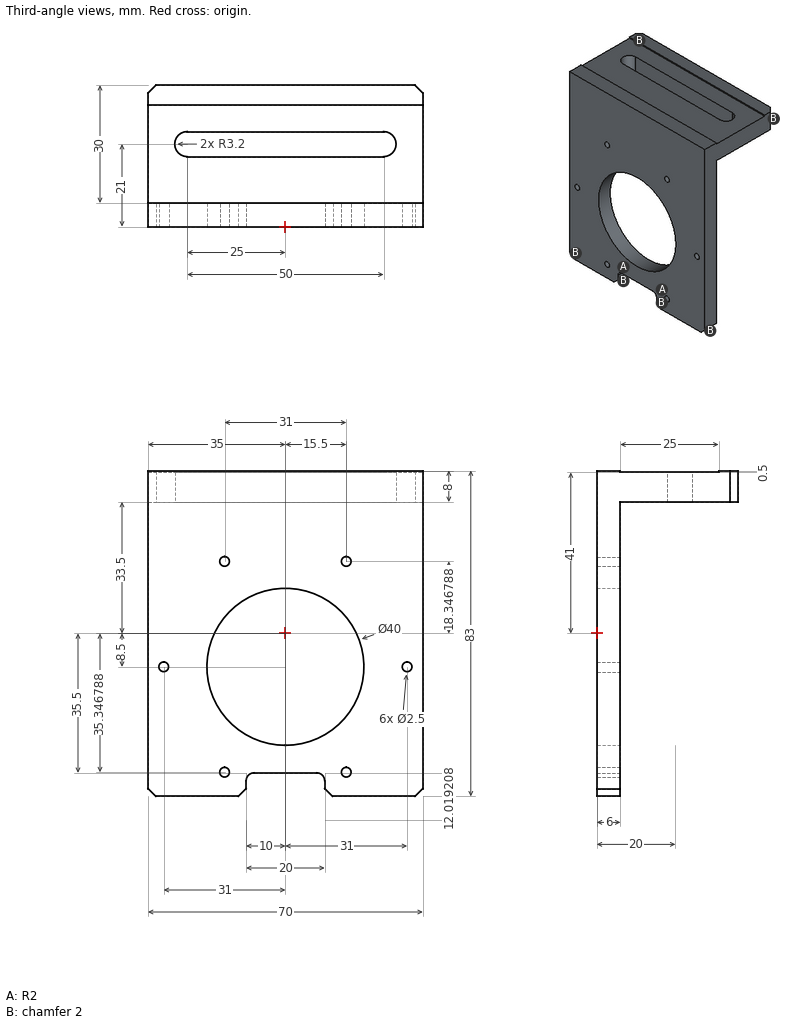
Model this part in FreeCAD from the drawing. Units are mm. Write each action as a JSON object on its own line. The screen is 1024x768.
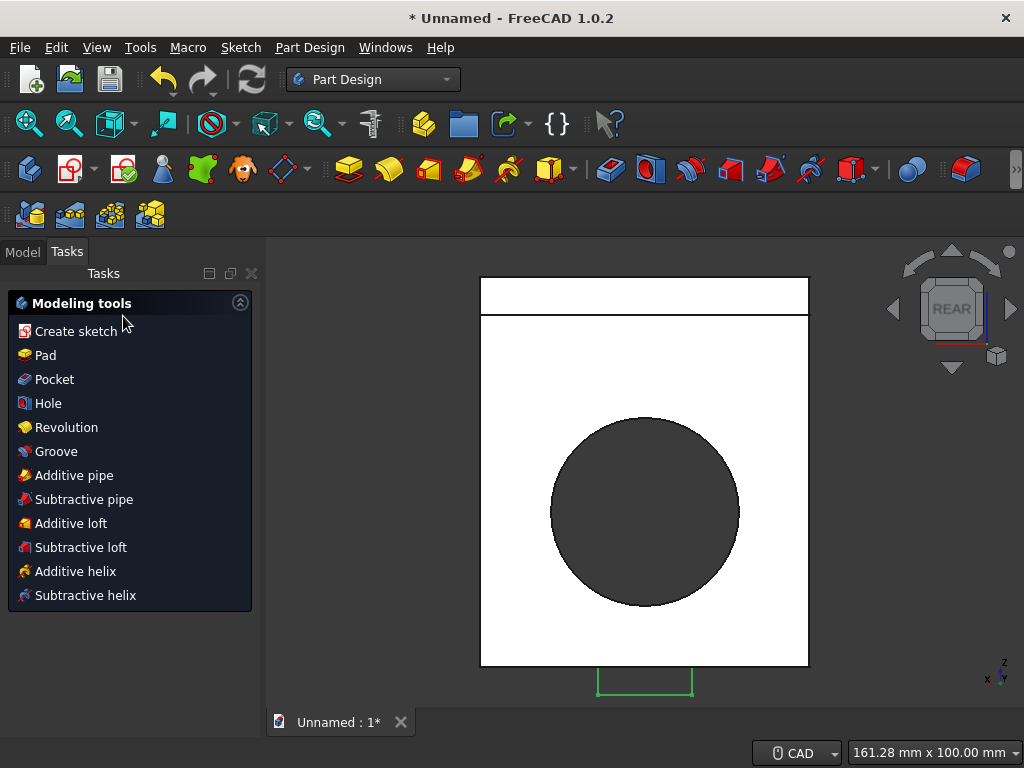
{"action": "left_click", "coordinate": [612, 170]}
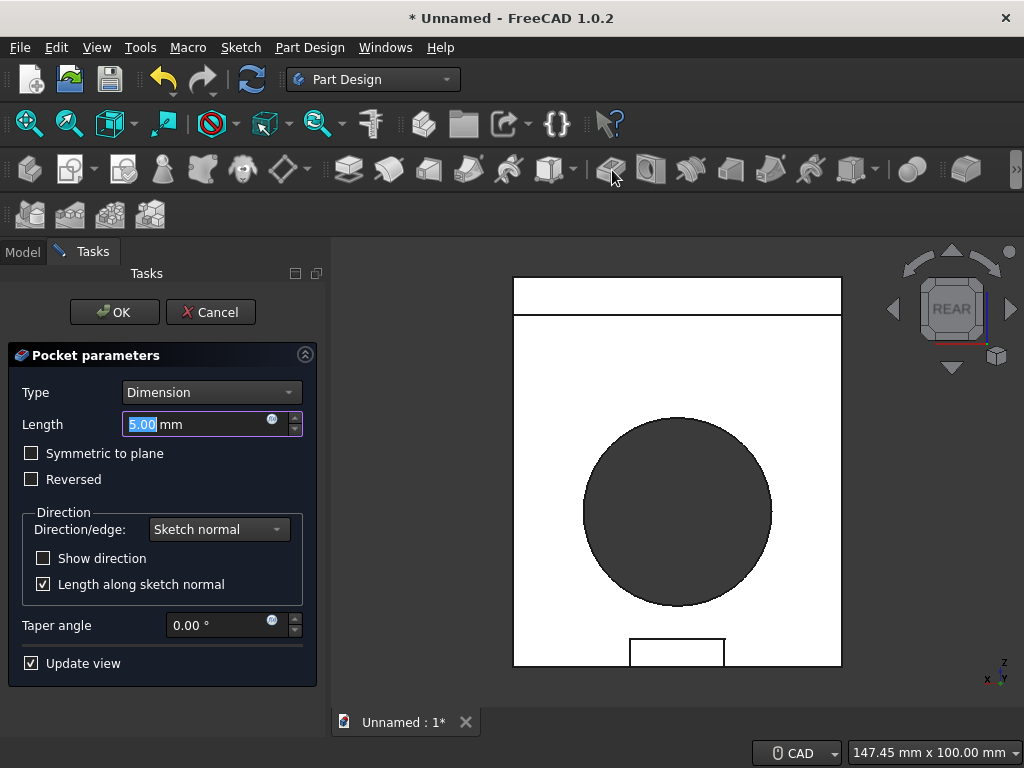
{"action": "type", "text": "20"}
{"action": "key", "text": "Tab"}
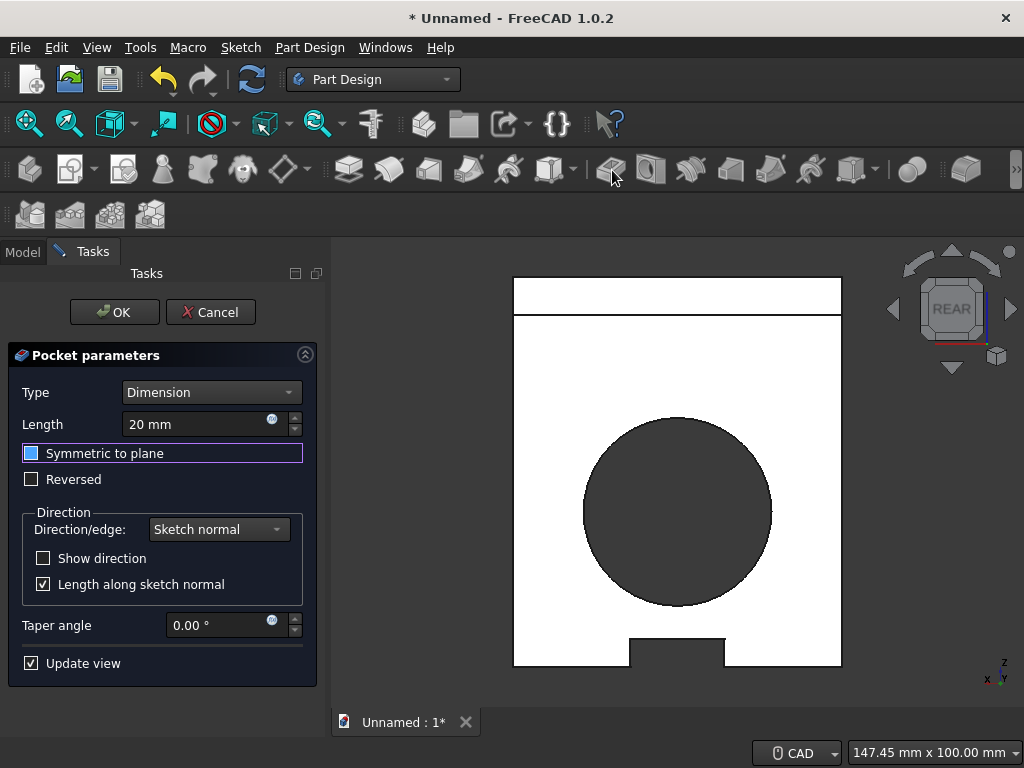
{"action": "left_click", "coordinate": [115, 312]}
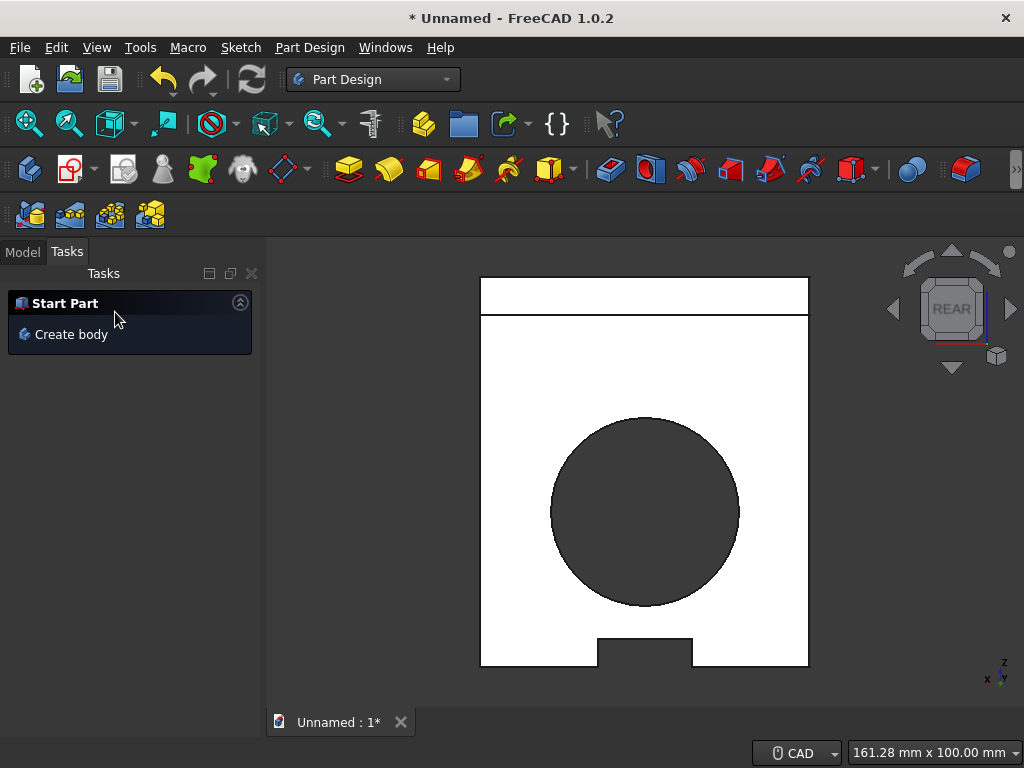
{"action": "left_click", "coordinate": [739, 389]}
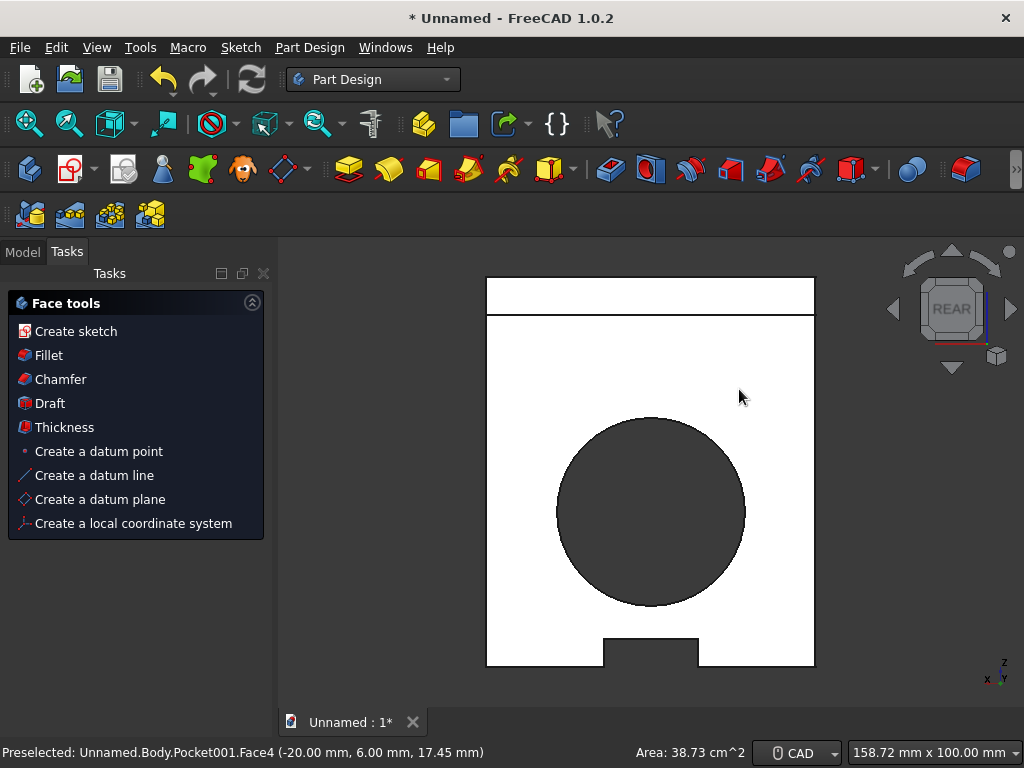
{"action": "left_click", "coordinate": [70, 170]}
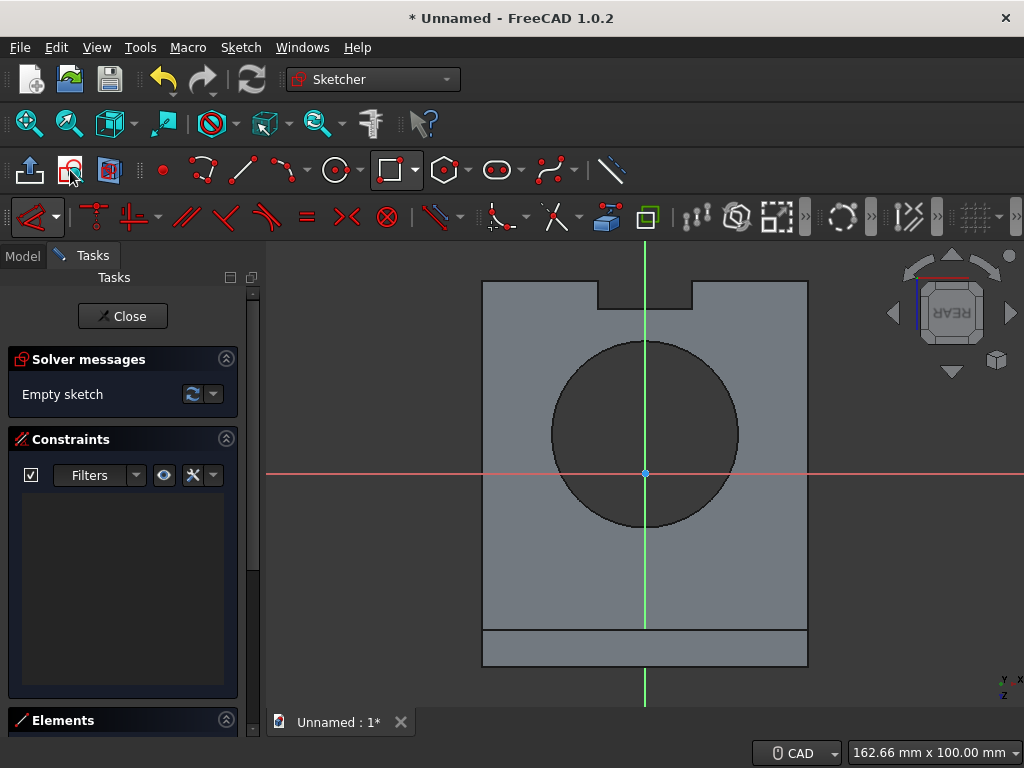
{"action": "left_click", "coordinate": [110, 170]}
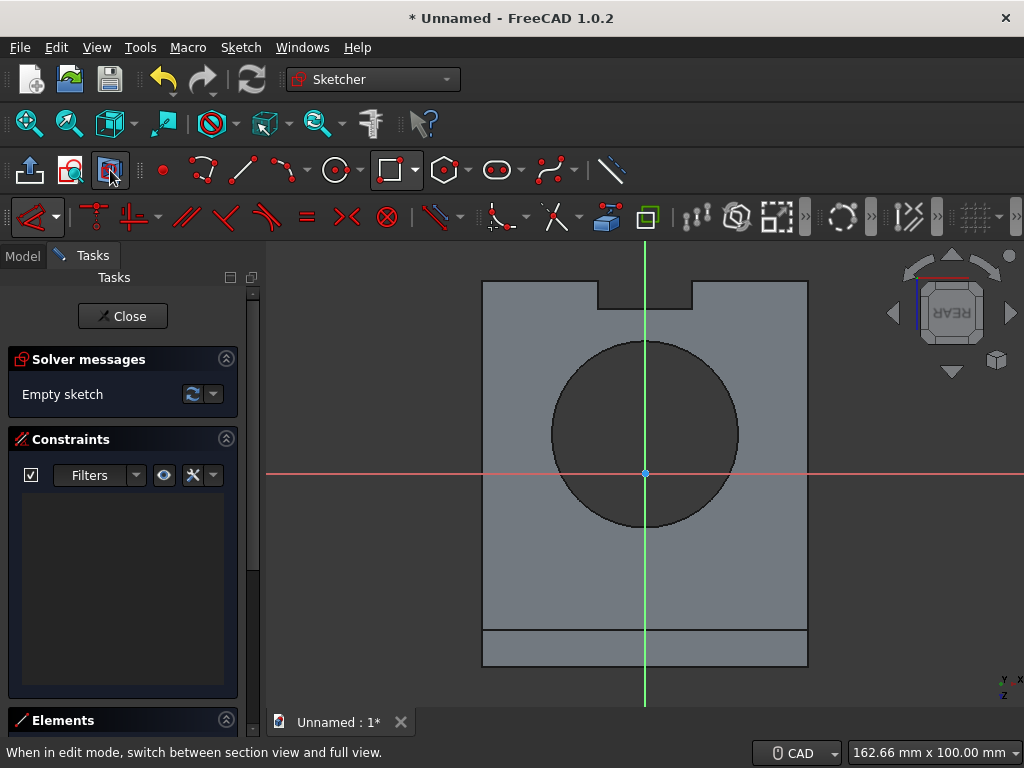
{"action": "left_click", "coordinate": [336, 170]}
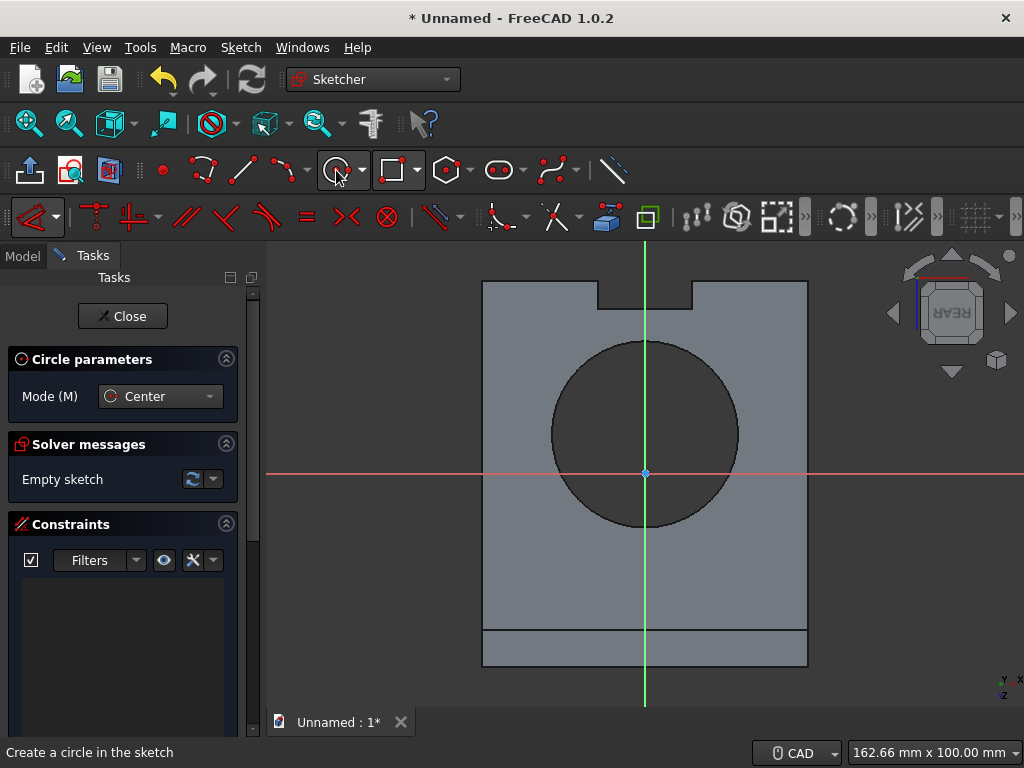
{"action": "scroll", "coordinate": [789, 434], "scroll_direction": "up", "scroll_amount": 7}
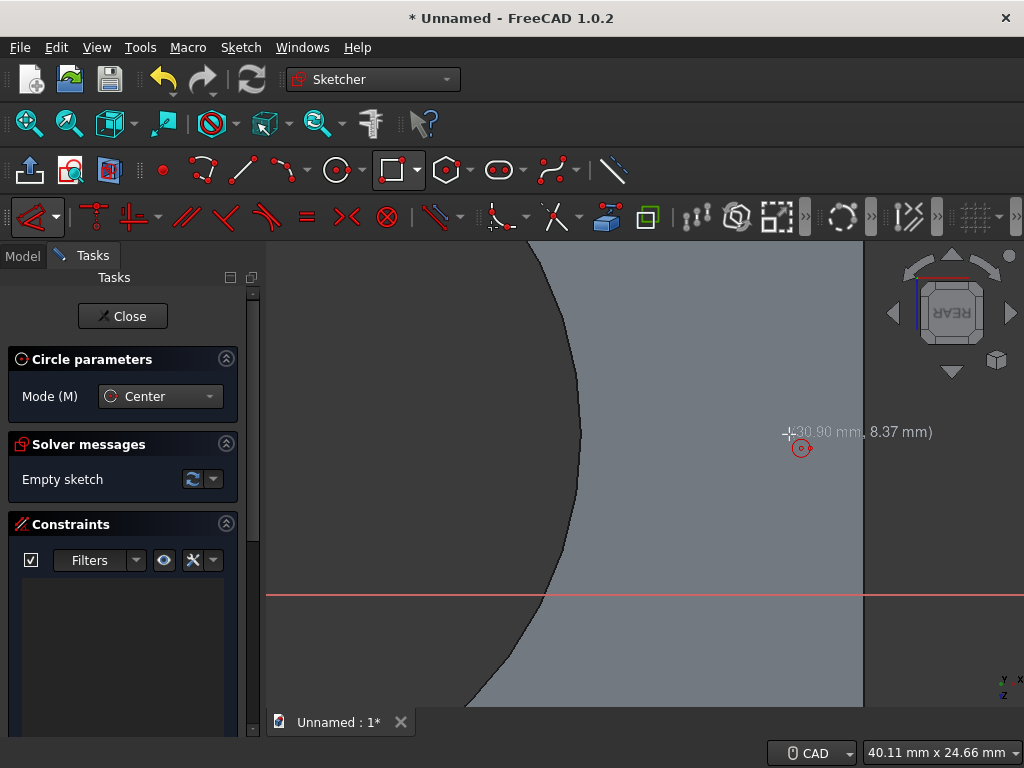
{"action": "scroll", "coordinate": [699, 487], "scroll_direction": "down", "scroll_amount": 7}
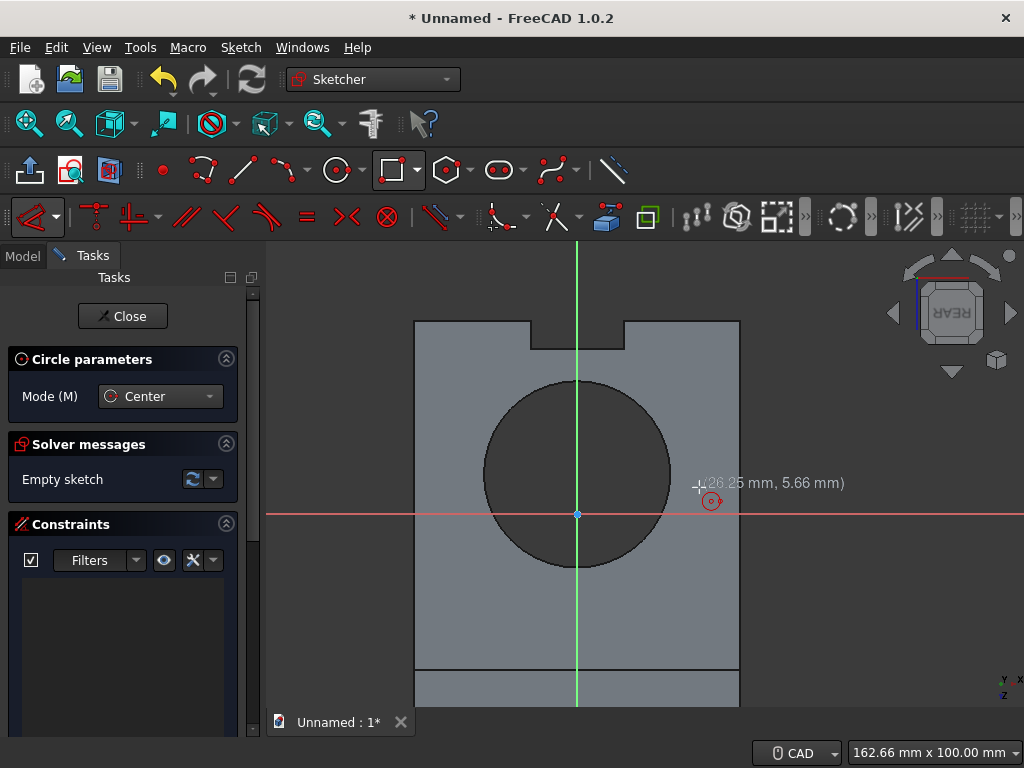
{"action": "left_click", "coordinate": [722, 474]}
{"action": "mouse_move", "coordinate": [726, 470]}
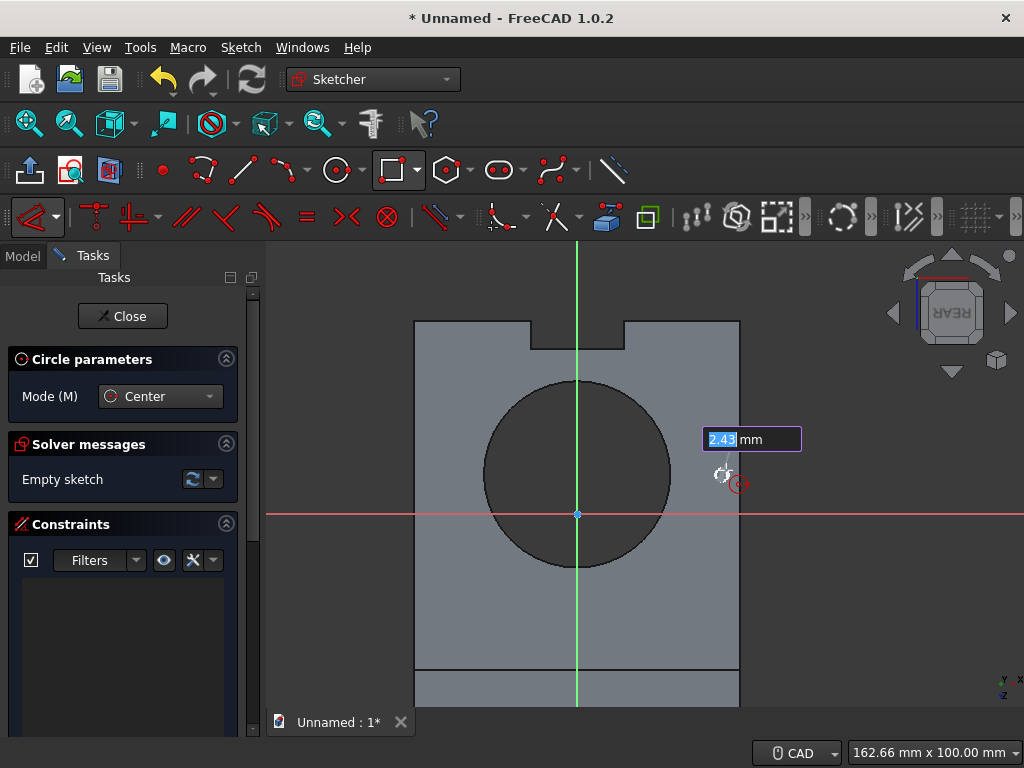
{"action": "type", "text": "2.5"}
{"action": "key", "text": "Return"}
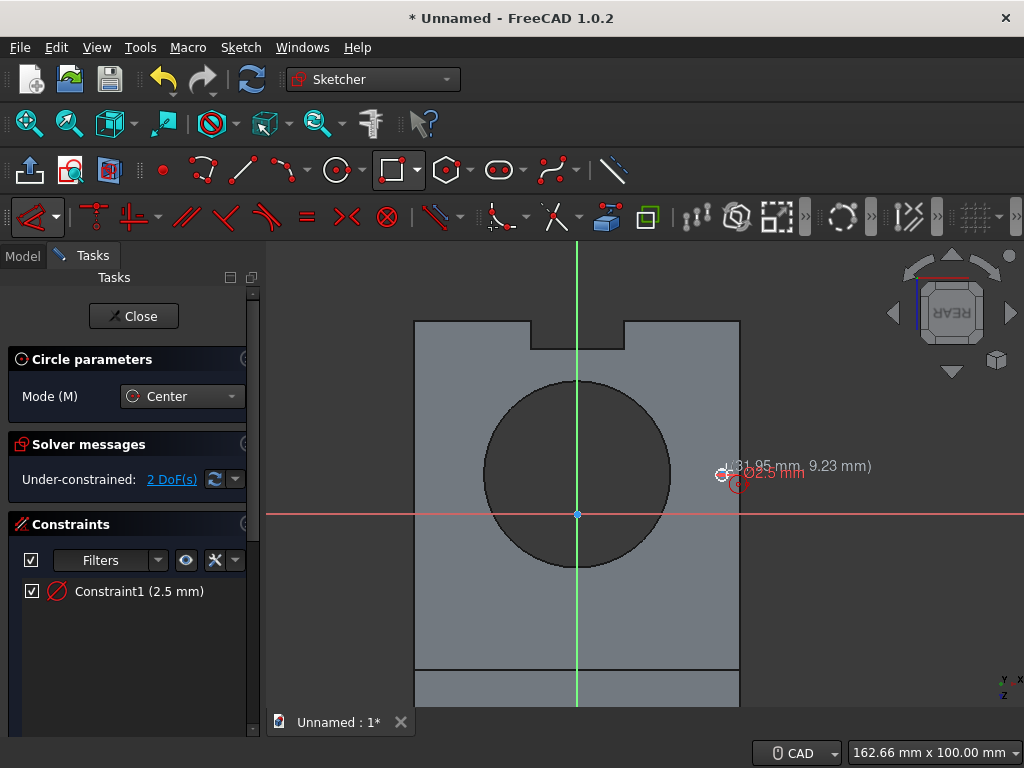
{"action": "scroll", "coordinate": [649, 600], "scroll_direction": "up", "scroll_amount": 7}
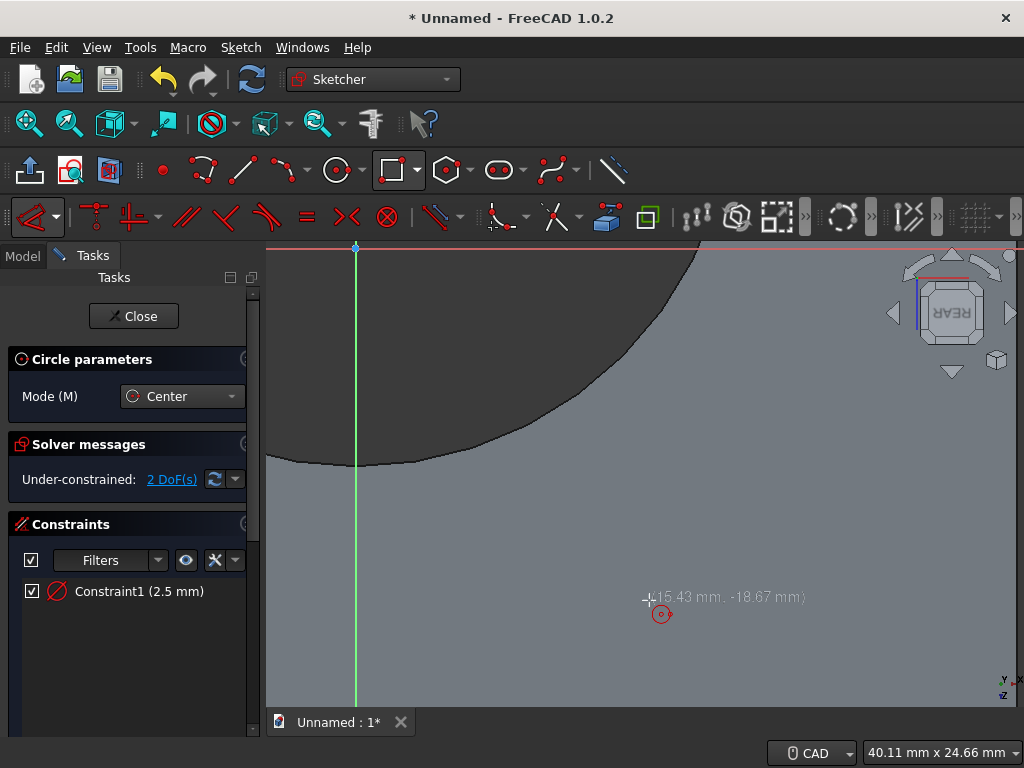
{"action": "scroll", "coordinate": [649, 600], "scroll_direction": "down", "scroll_amount": 7}